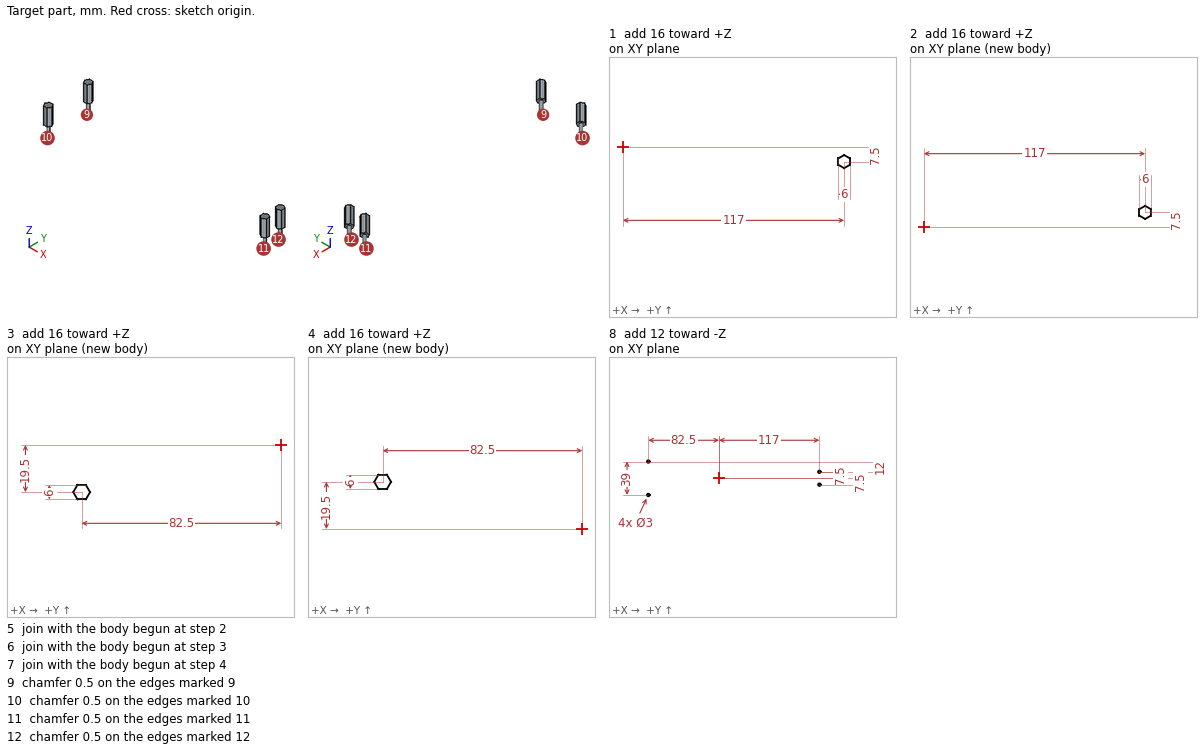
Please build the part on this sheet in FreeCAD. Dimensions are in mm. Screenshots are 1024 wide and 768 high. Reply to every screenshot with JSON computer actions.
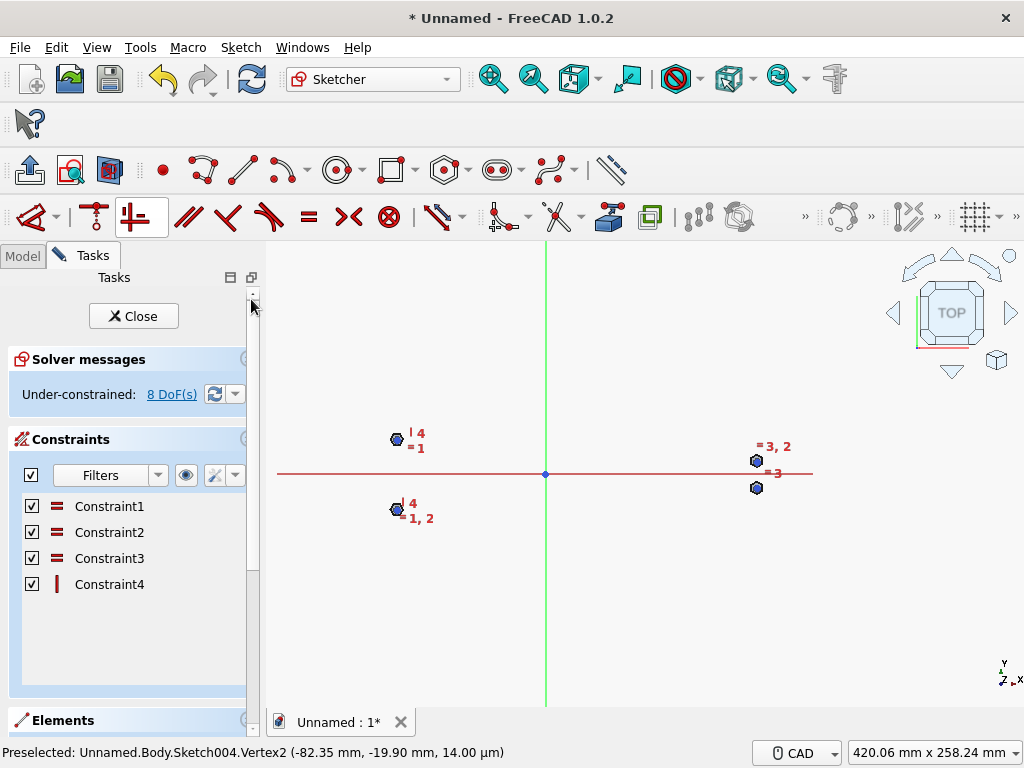
{"action": "left_click", "coordinate": [757, 462]}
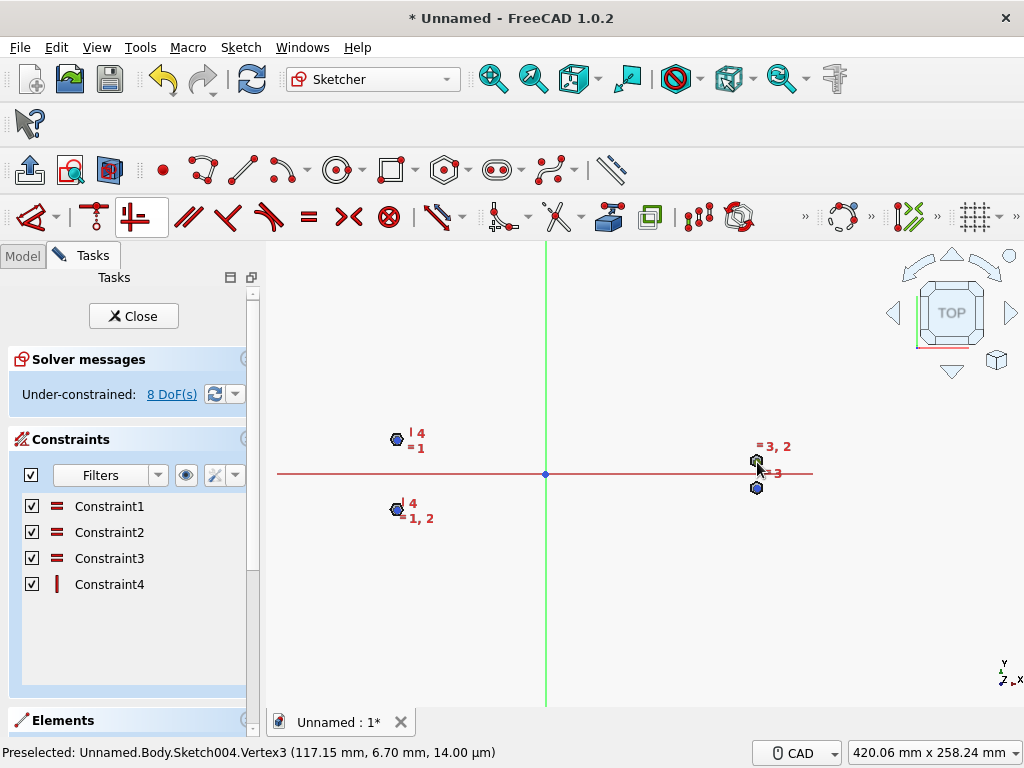
{"action": "left_click", "coordinate": [757, 489]}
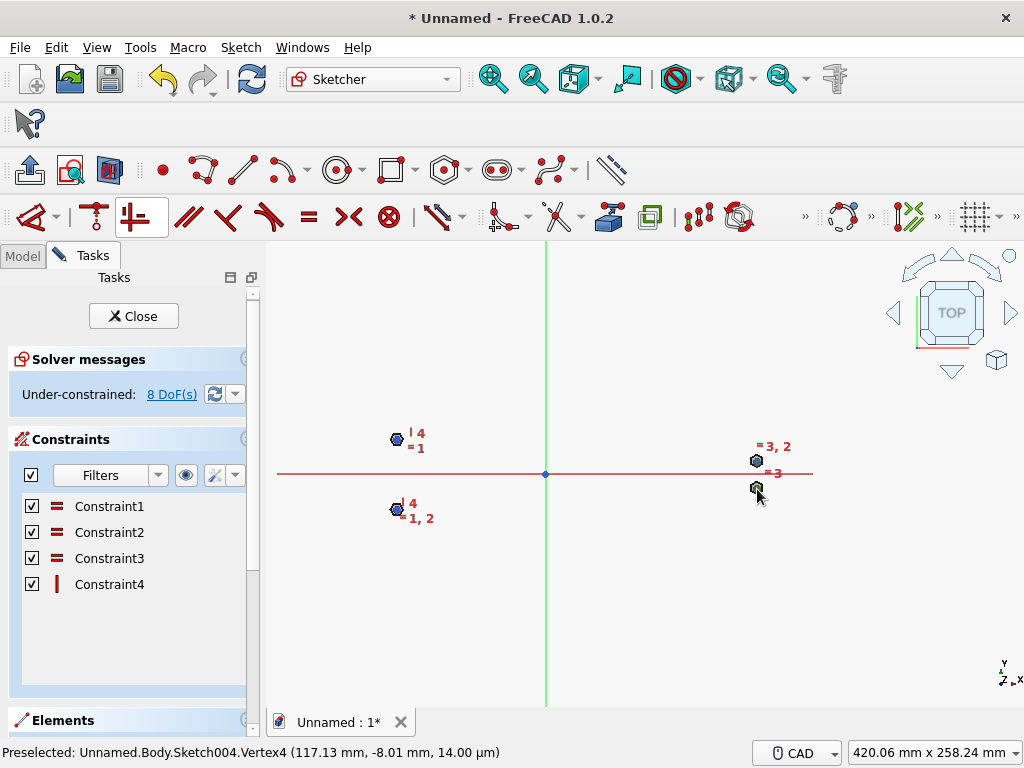
{"action": "left_click", "coordinate": [162, 218]}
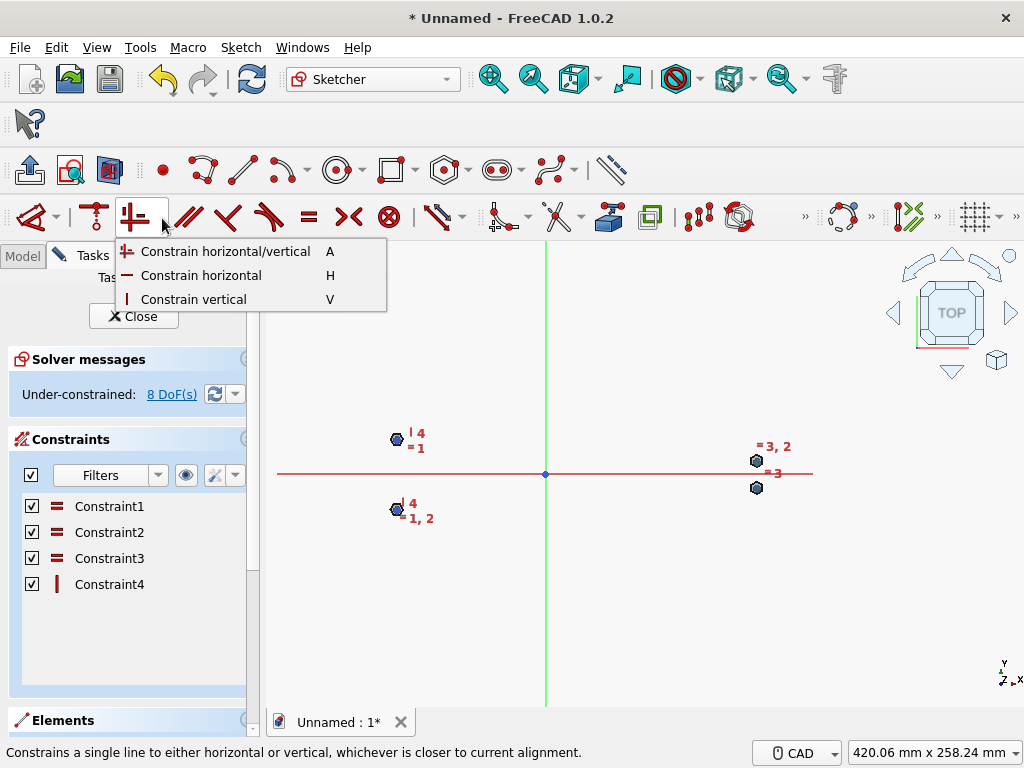
{"action": "left_click", "coordinate": [251, 299]}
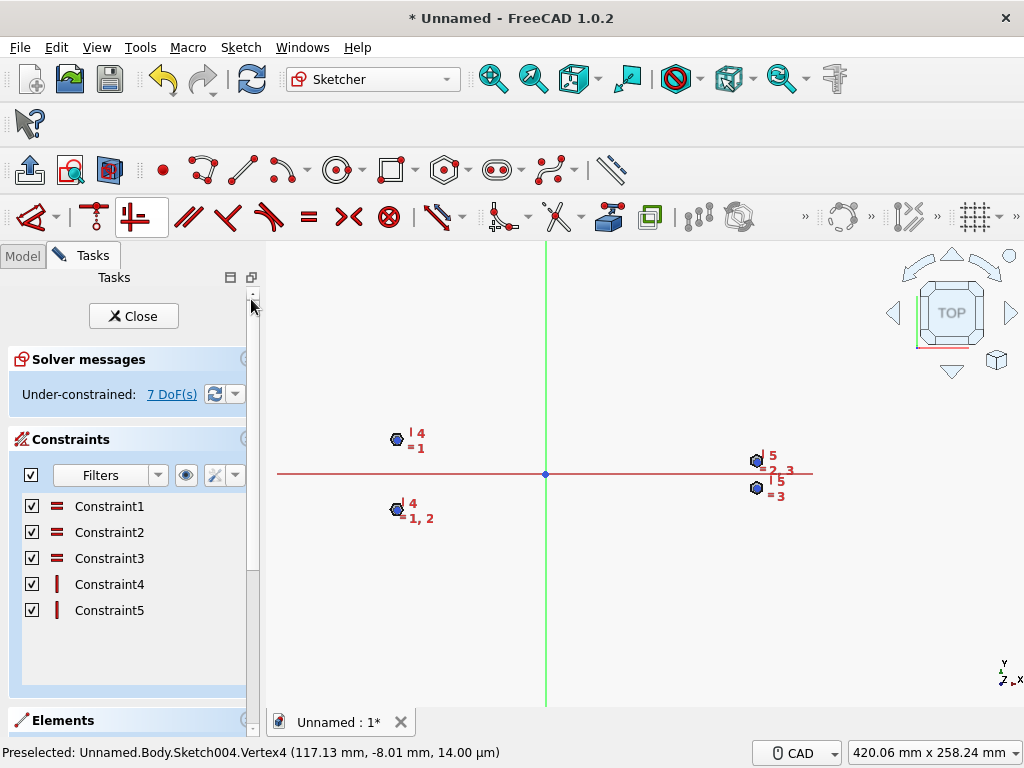
{"action": "left_click", "coordinate": [32, 218]}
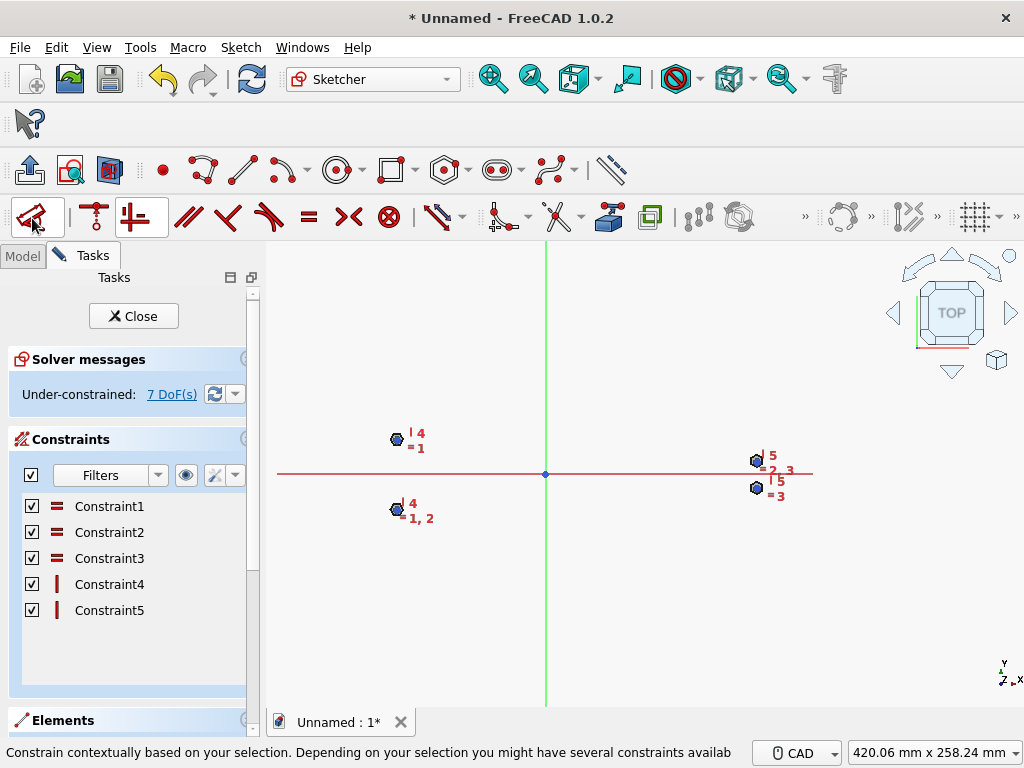
{"action": "scroll", "coordinate": [399, 438], "scroll_direction": "up", "scroll_amount": 10}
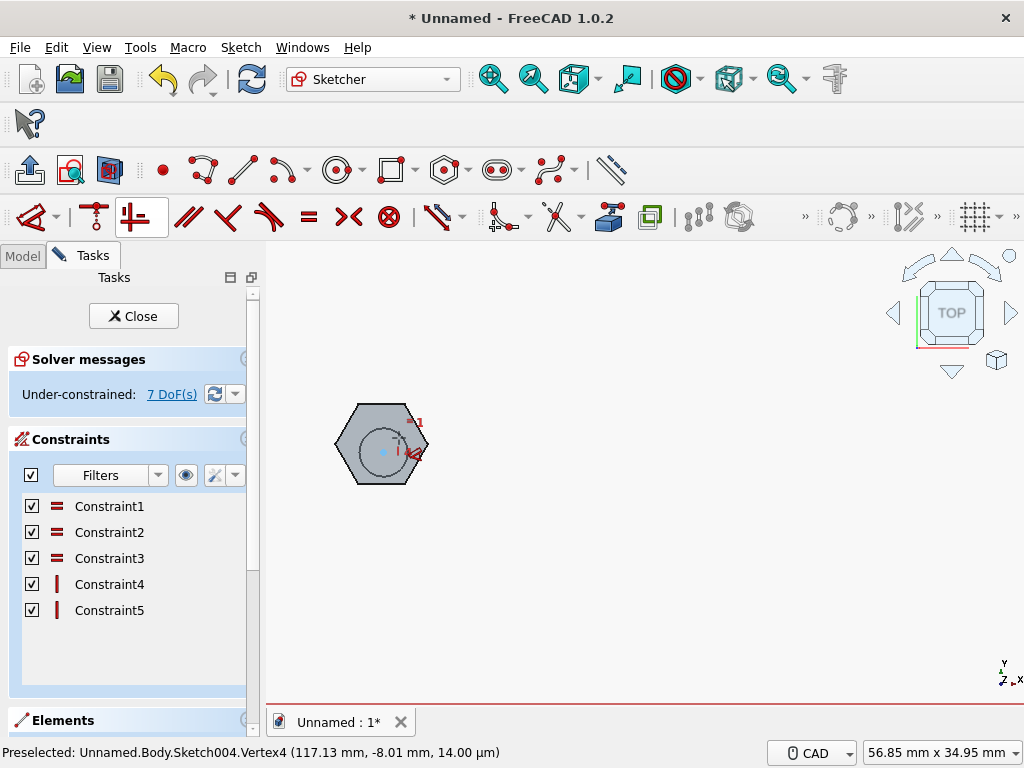
{"action": "left_click", "coordinate": [401, 435]}
{"action": "left_click", "coordinate": [424, 412]}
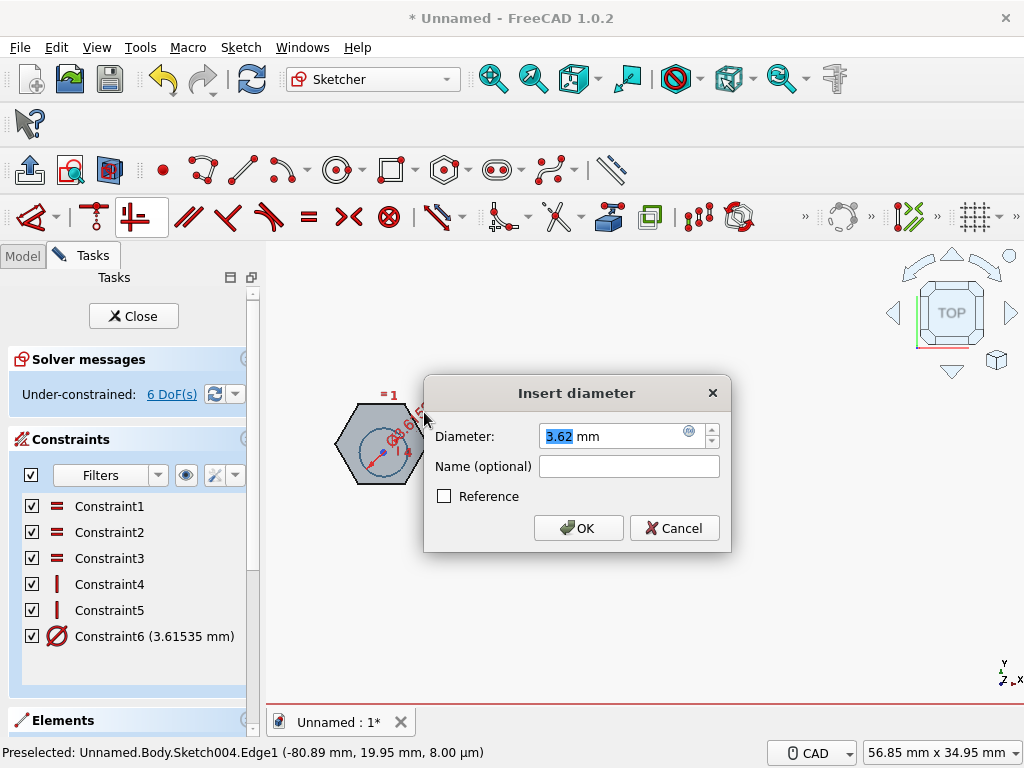
{"action": "type", "text": "3"}
{"action": "key", "text": "Return"}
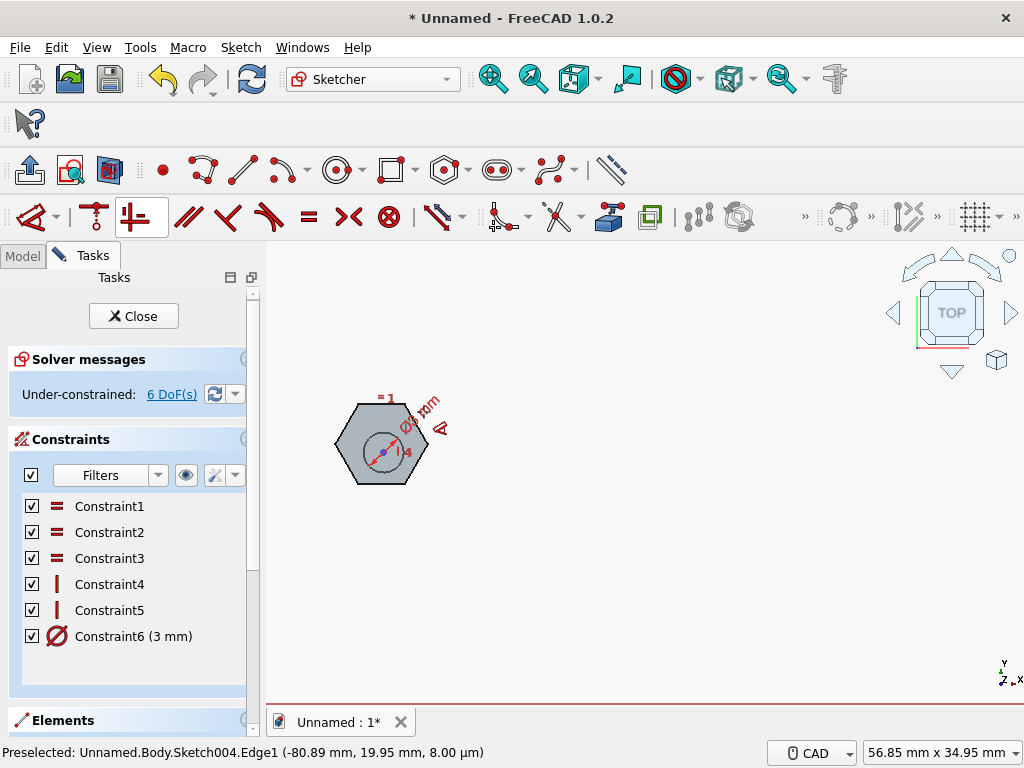
{"action": "scroll", "coordinate": [399, 438], "scroll_direction": "down", "scroll_amount": 10}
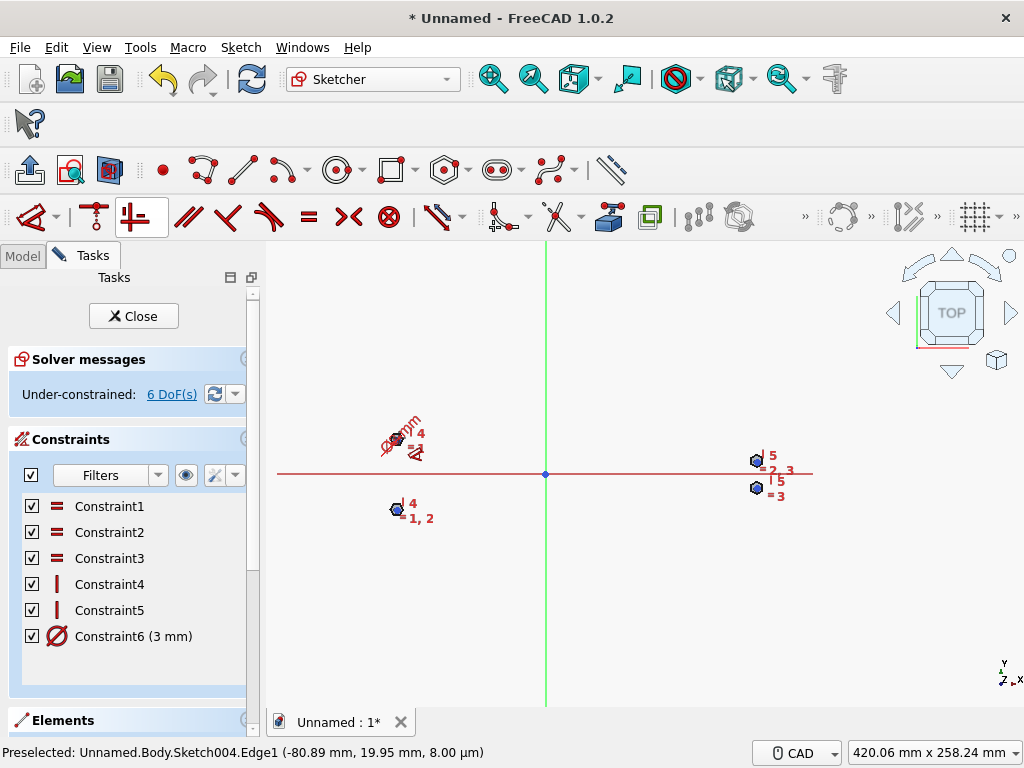
{"action": "left_click", "coordinate": [757, 462]}
{"action": "left_click", "coordinate": [651, 428]}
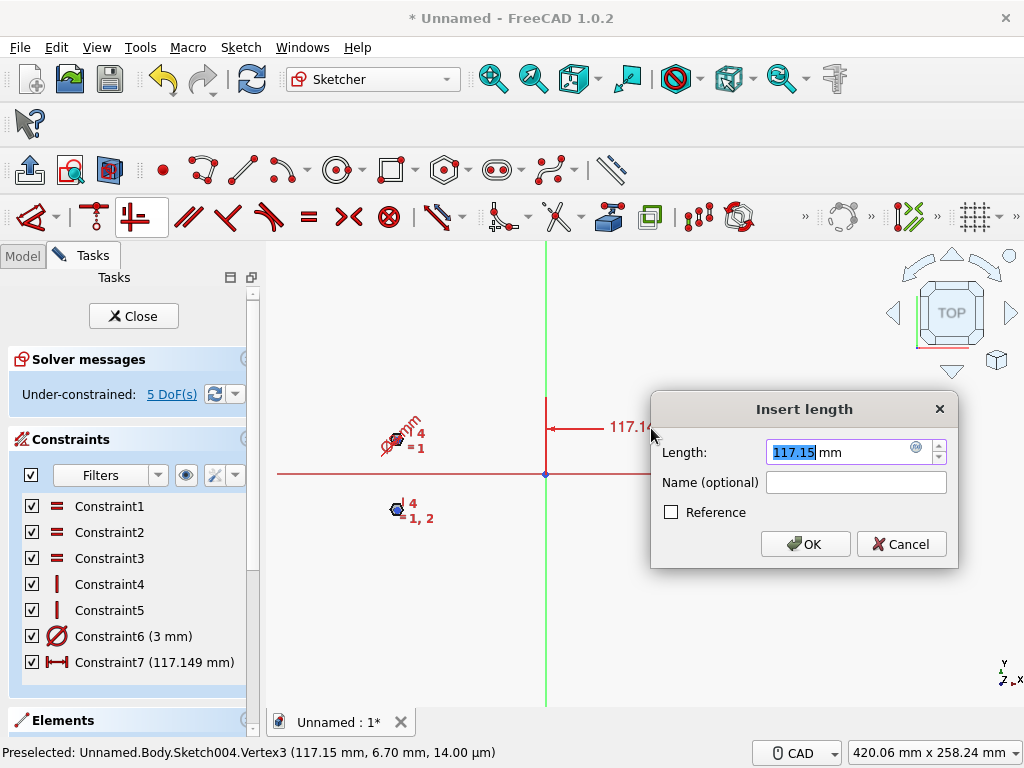
{"action": "type", "text": "117"}
{"action": "key", "text": "Return"}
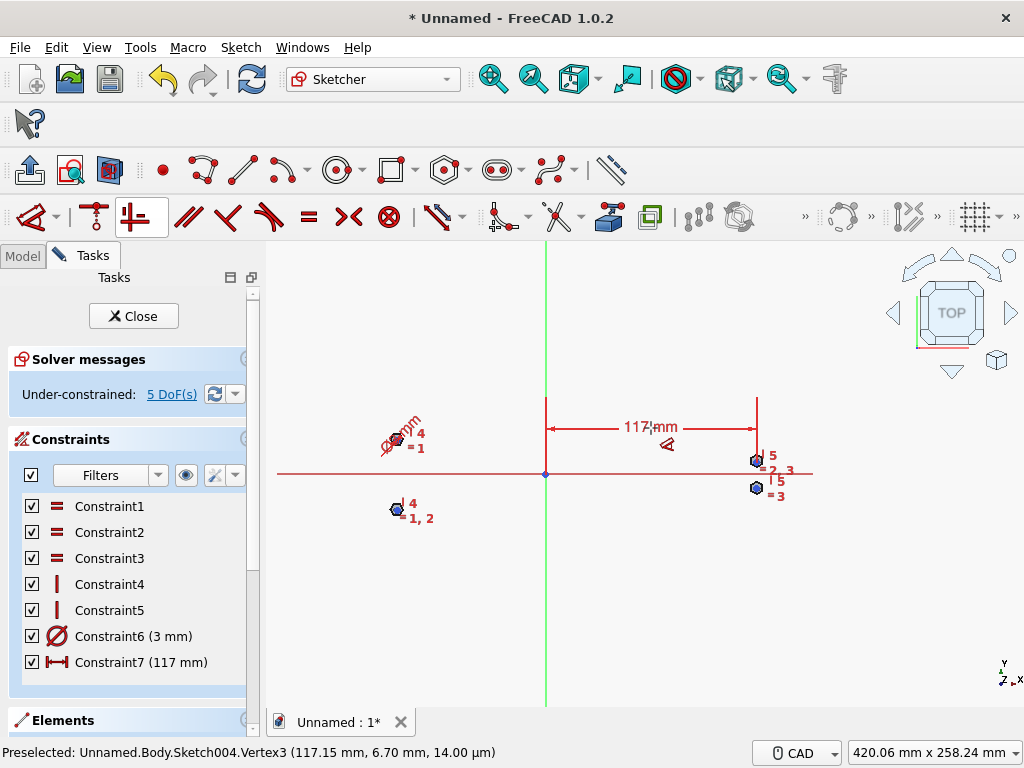
{"action": "scroll", "coordinate": [757, 462], "scroll_direction": "up", "scroll_amount": 6}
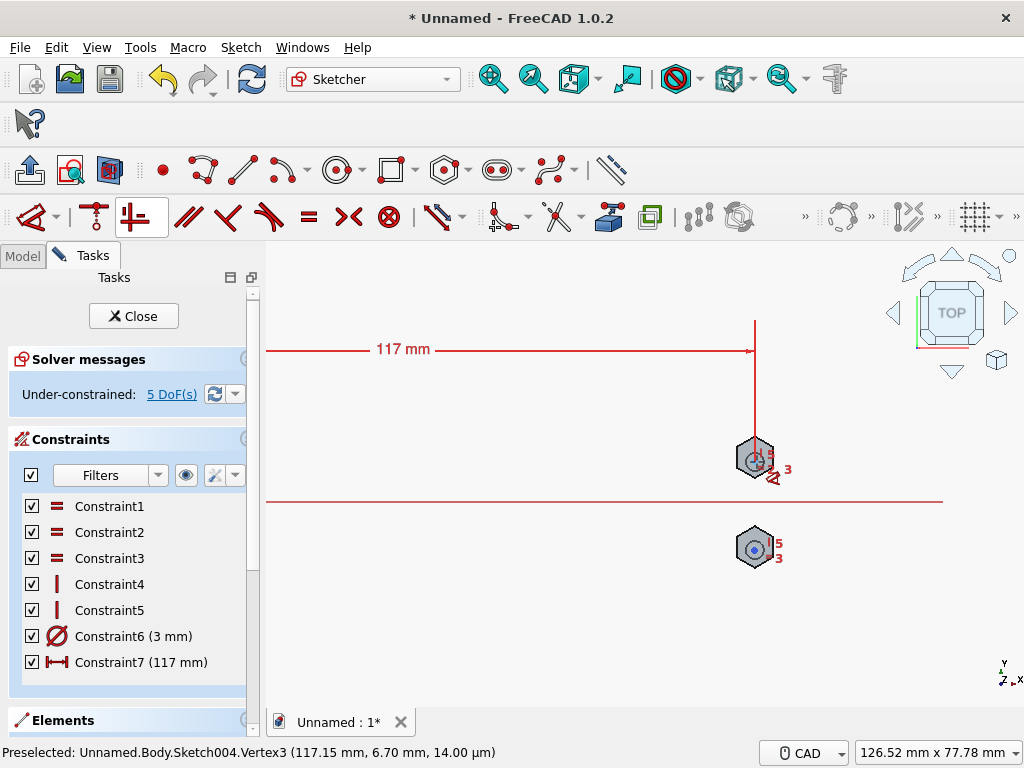
{"action": "left_click", "coordinate": [755, 462]}
{"action": "left_click", "coordinate": [789, 482]}